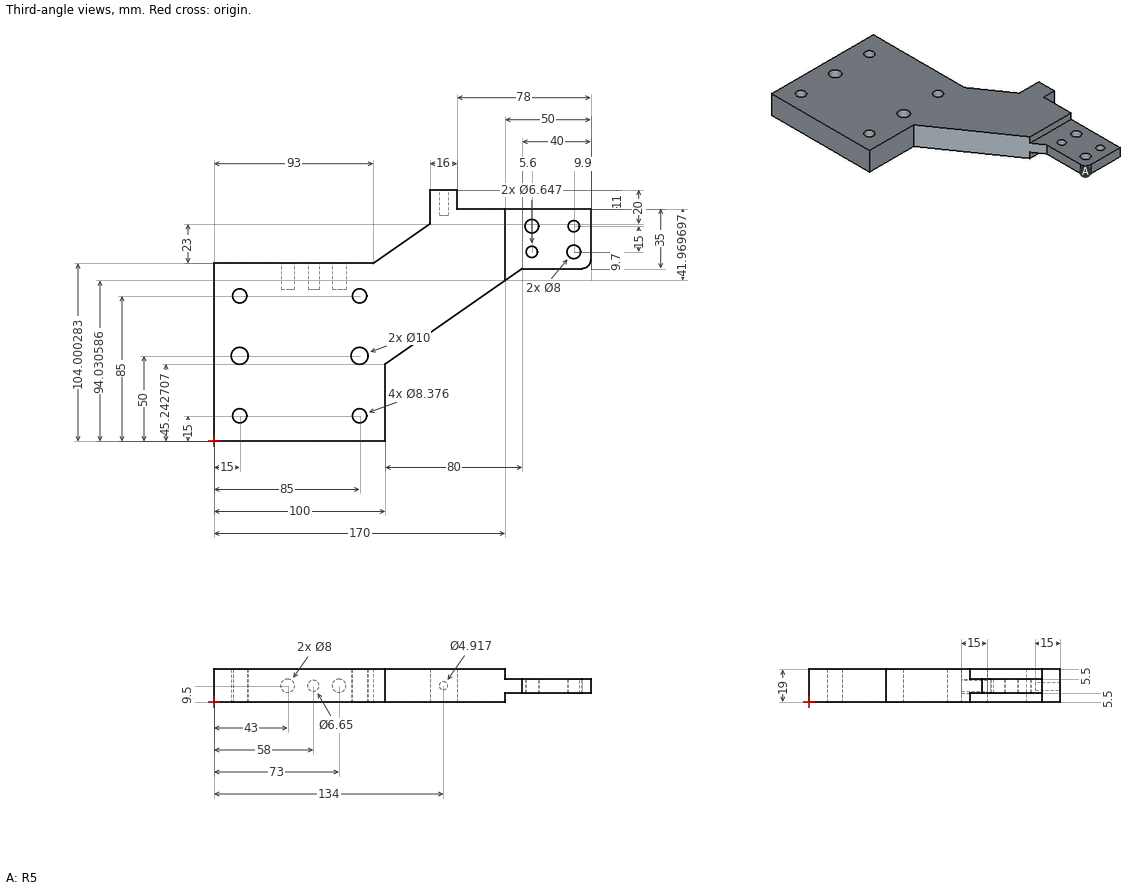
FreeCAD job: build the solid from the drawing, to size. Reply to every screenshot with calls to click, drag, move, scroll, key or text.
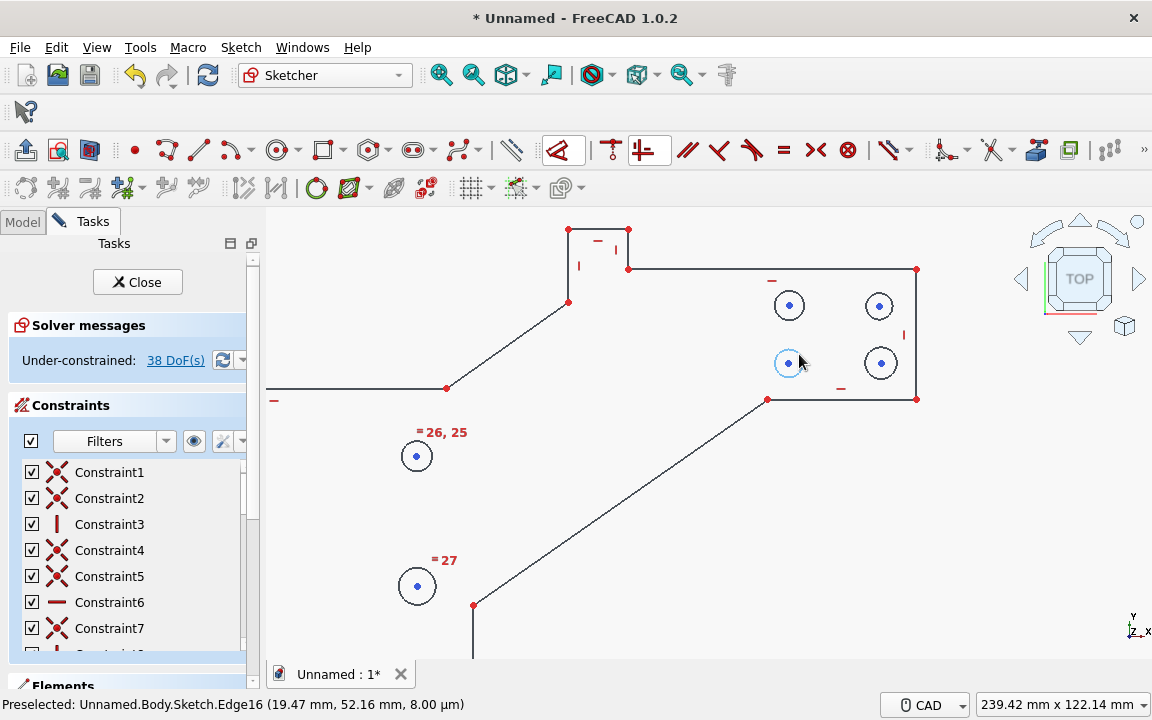
click(799, 354)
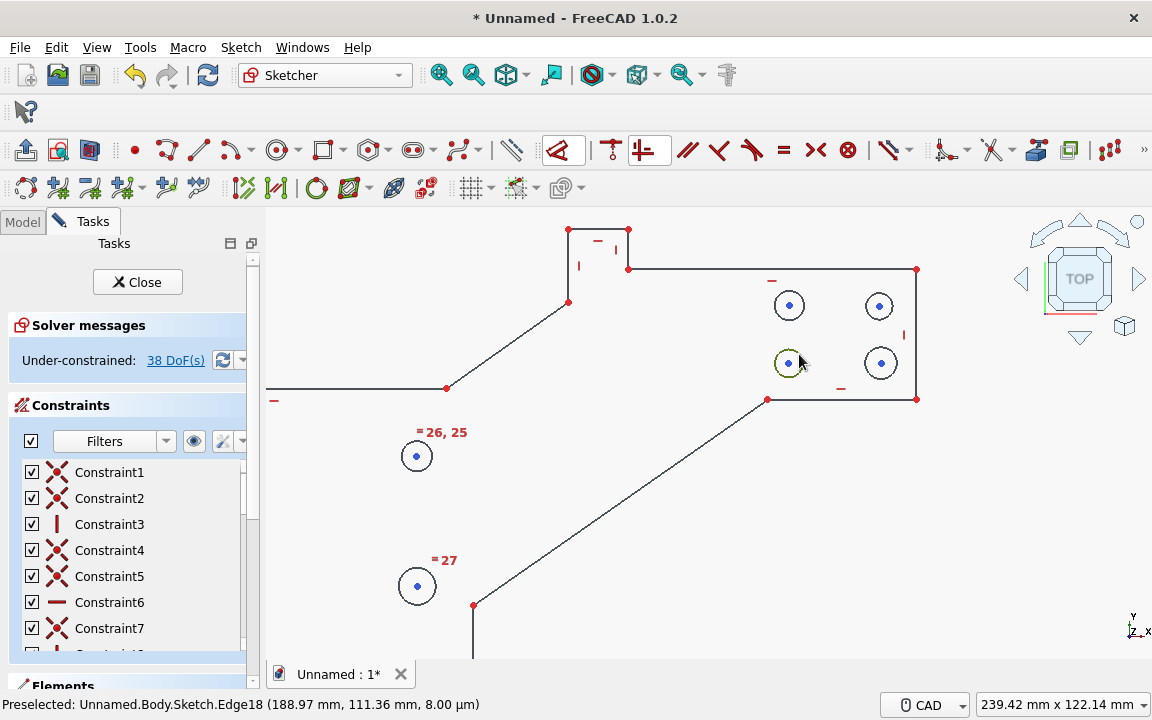
click(889, 297)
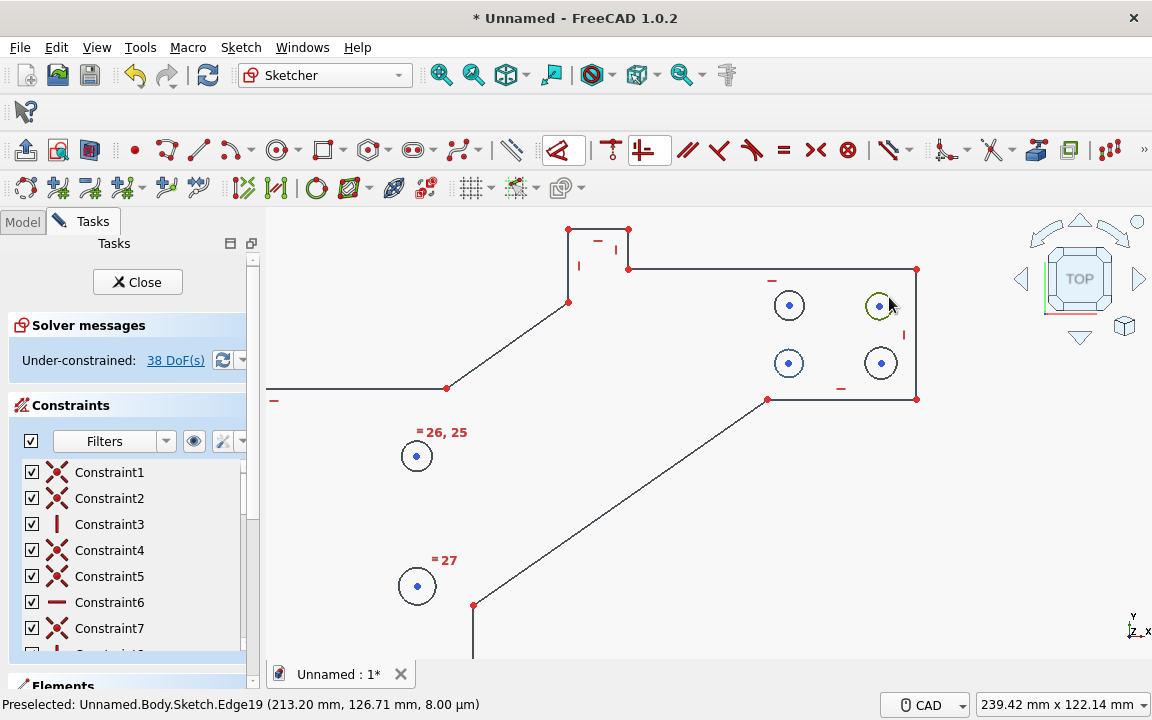
click(784, 150)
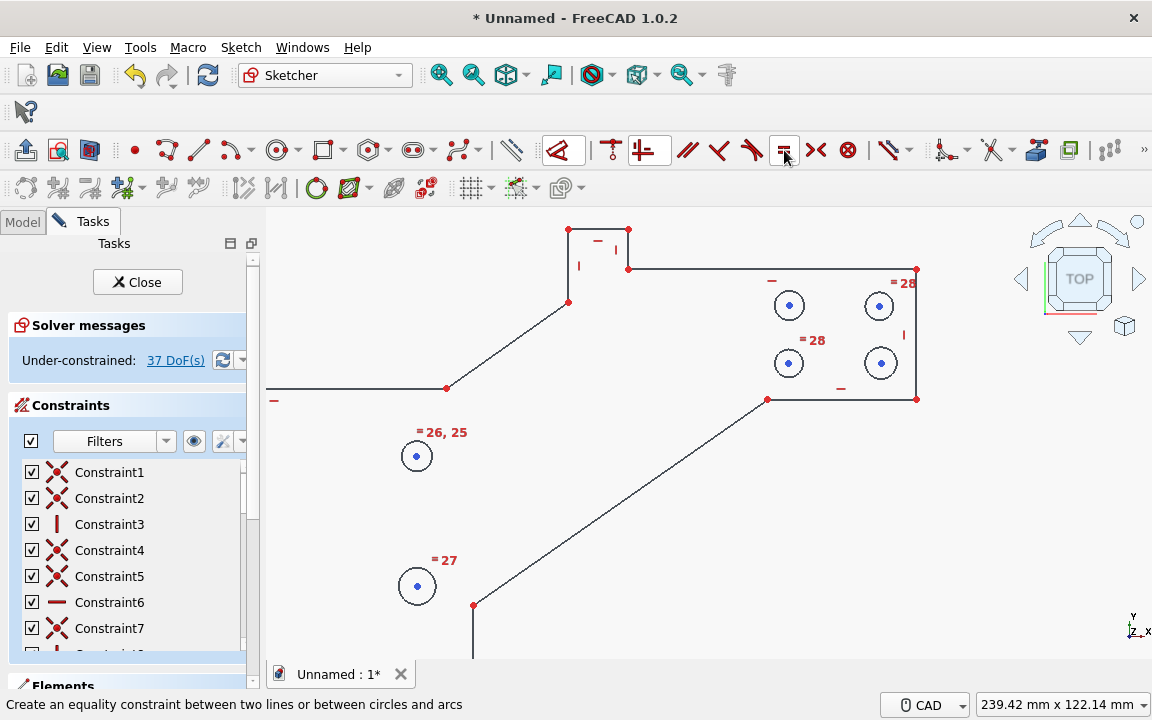
click(892, 352)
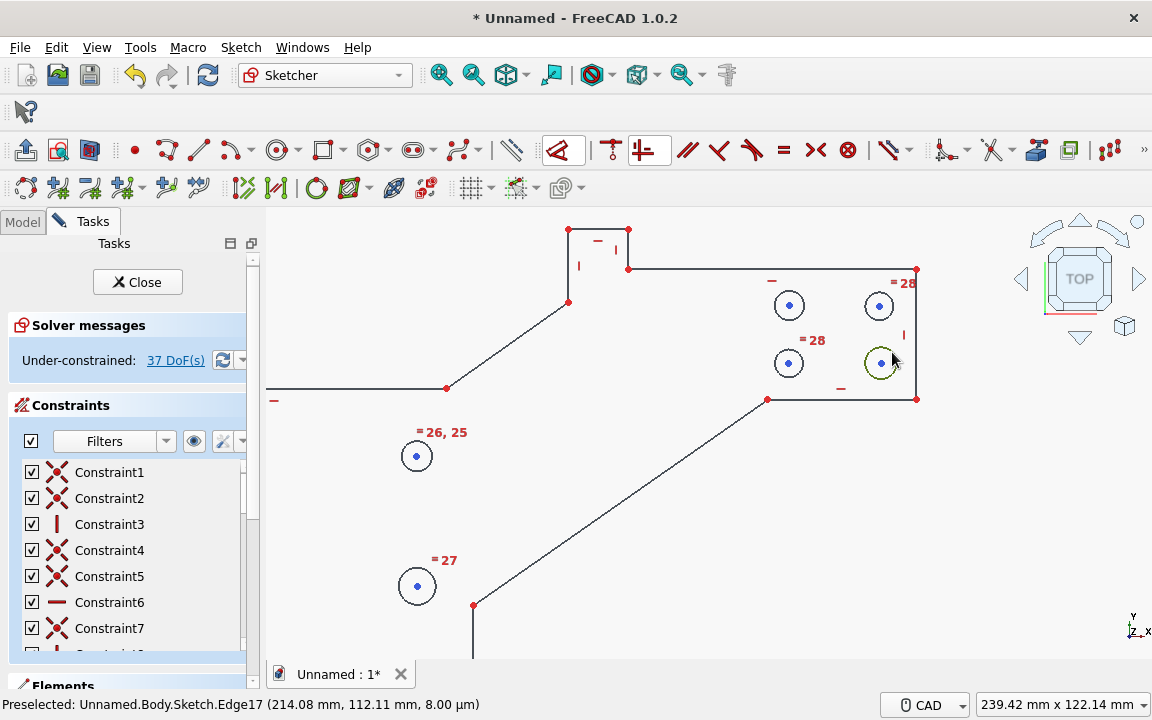
click(800, 295)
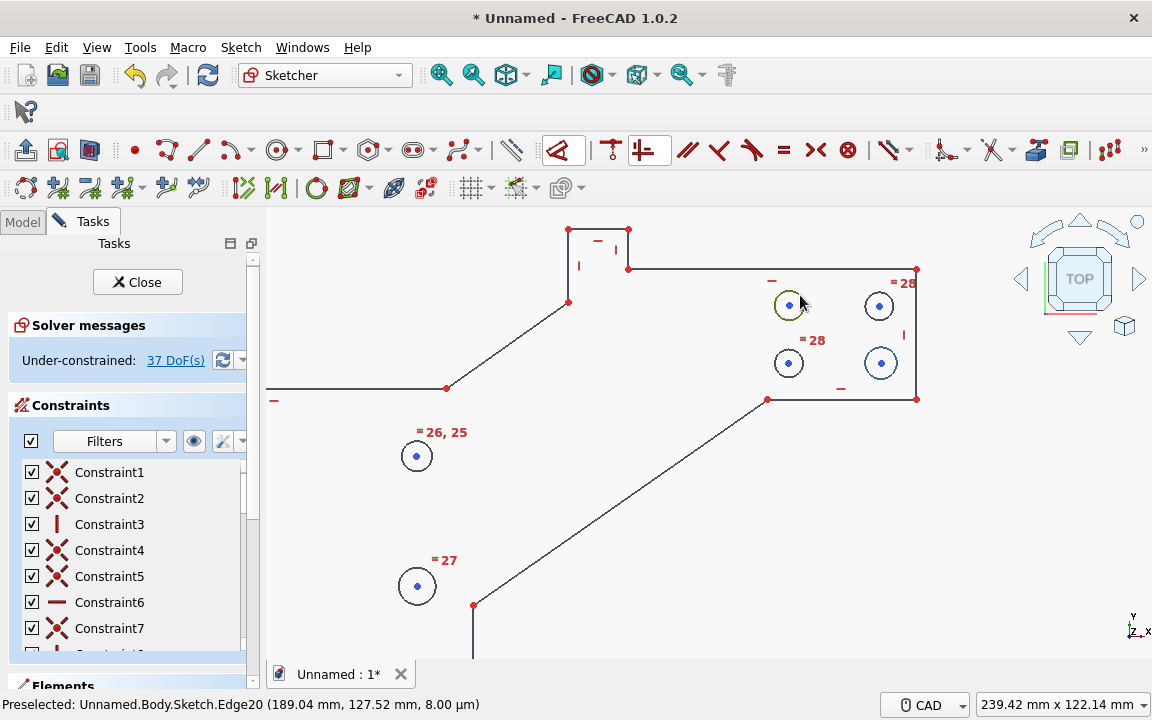
click(784, 150)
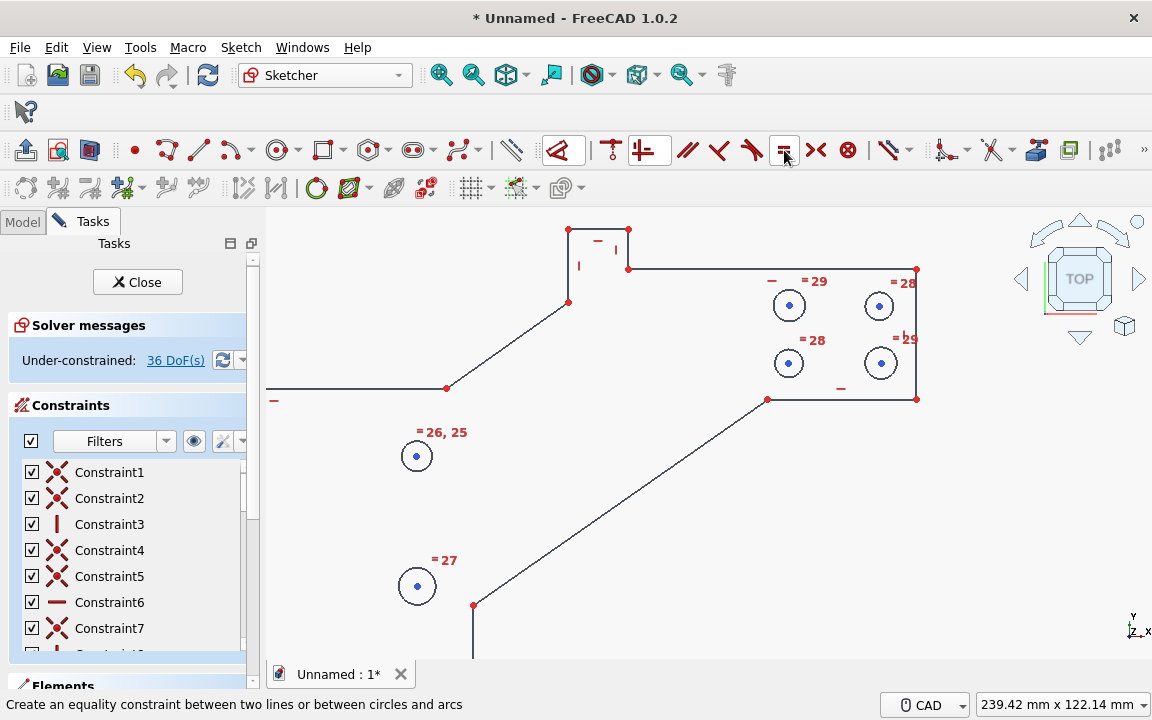
click(558, 150)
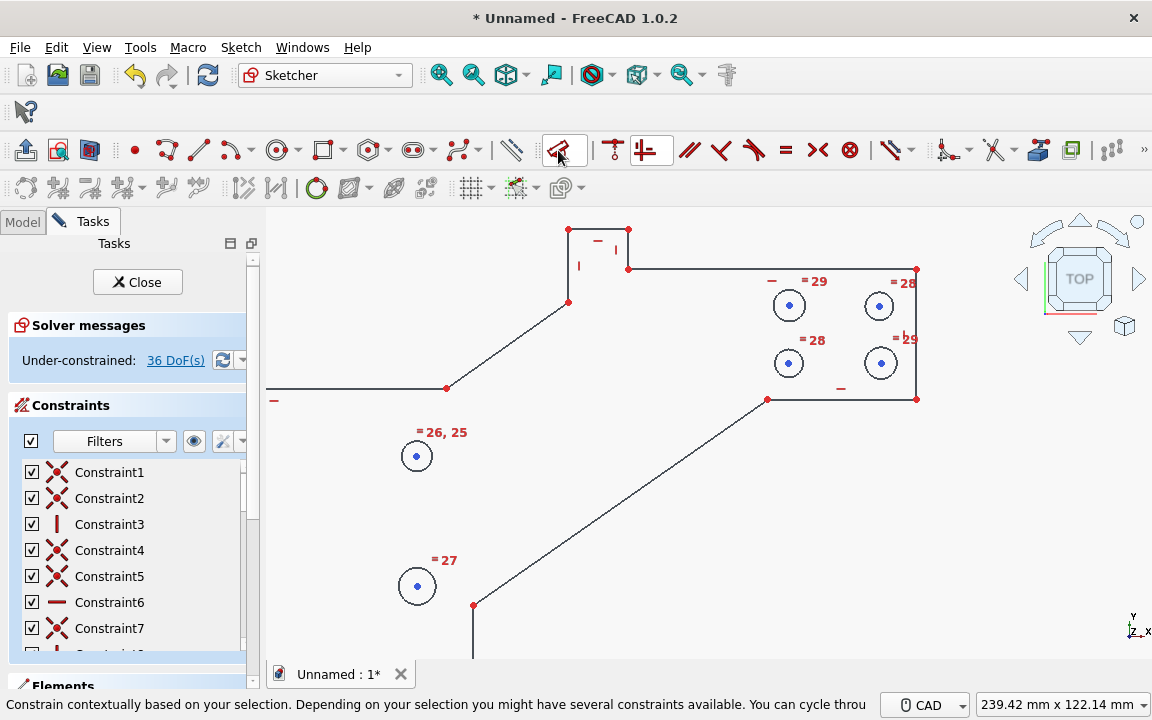
scroll(800, 353, down, 3)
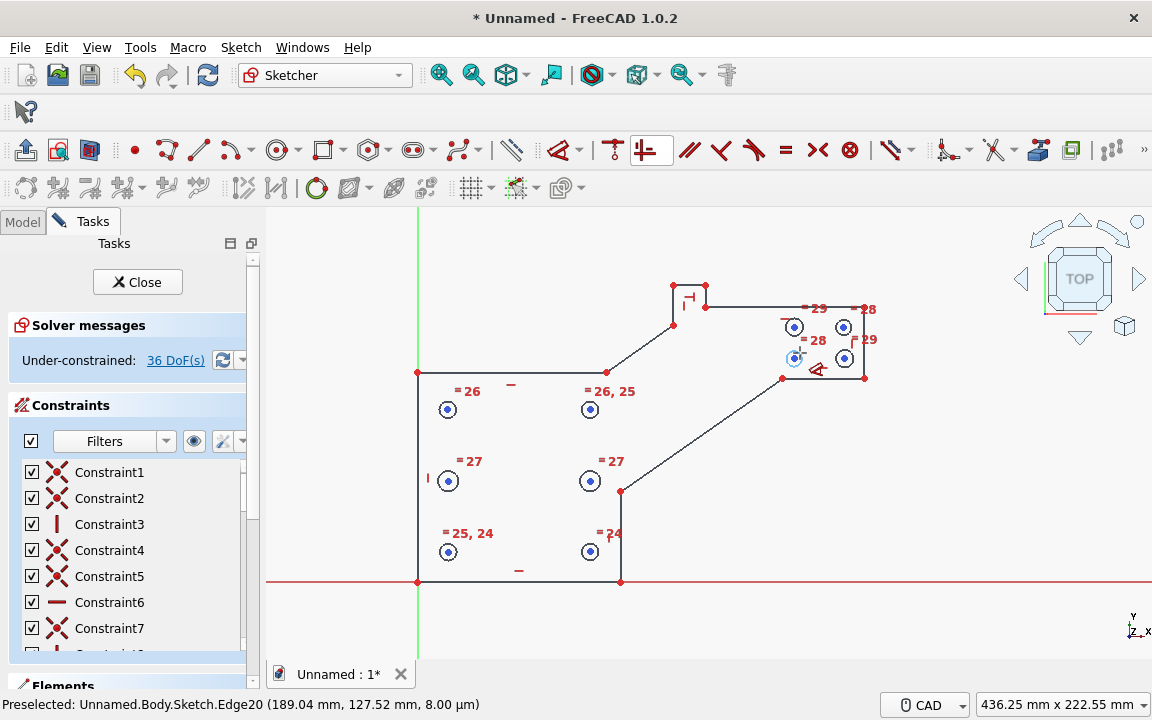
scroll(596, 546, up, 5)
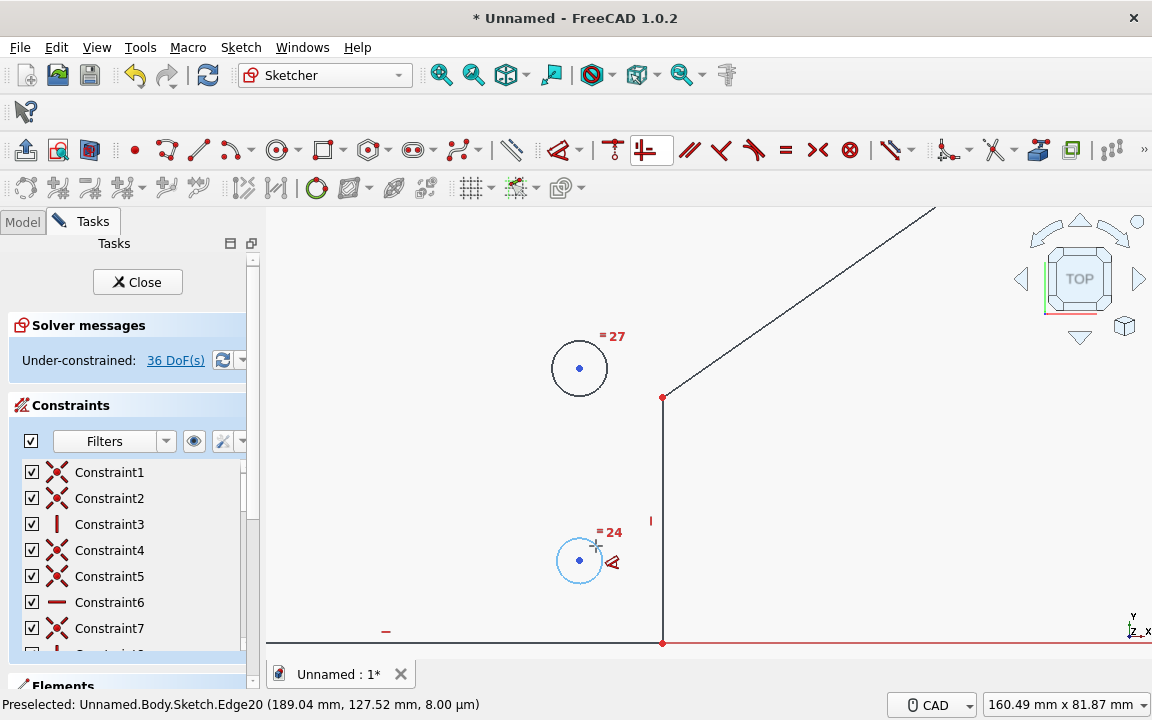
click(595, 545)
click(617, 522)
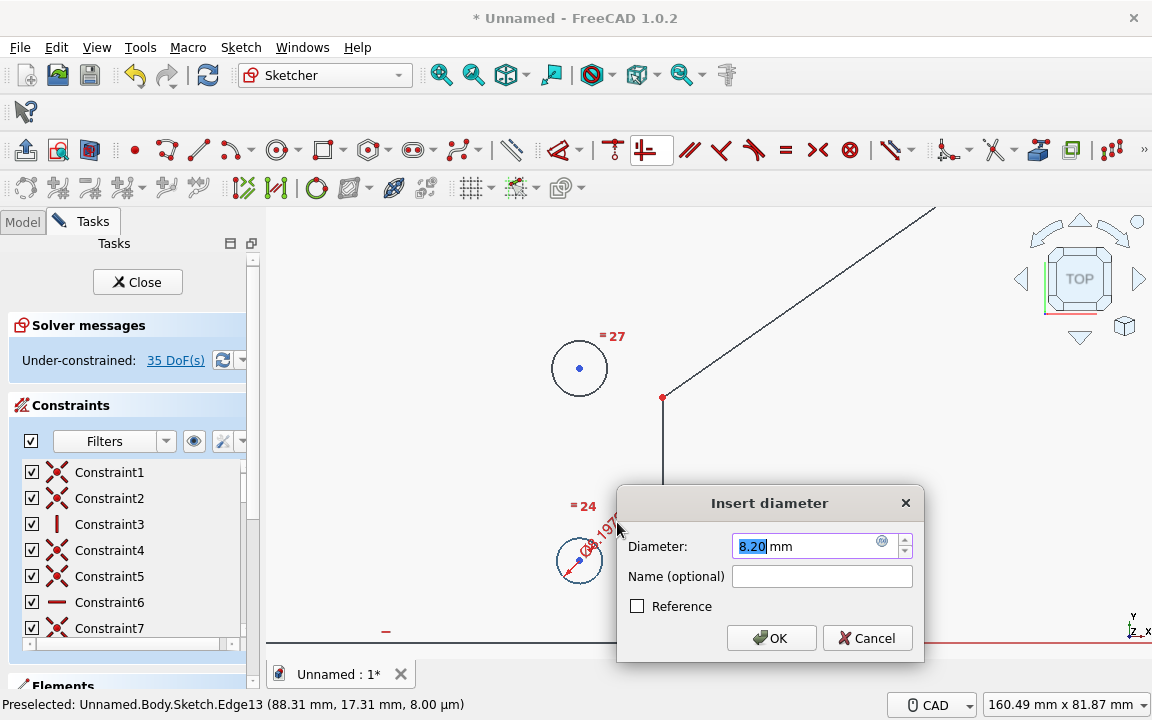
text(8.376)
key(Return)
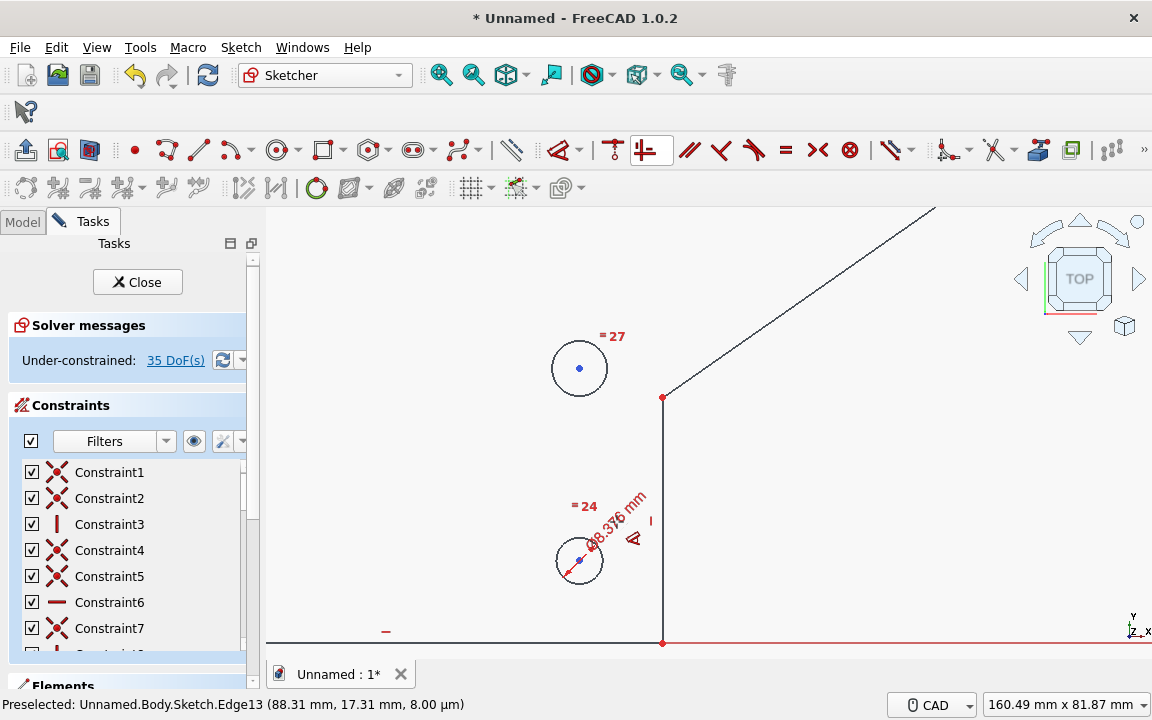
click(599, 349)
click(622, 326)